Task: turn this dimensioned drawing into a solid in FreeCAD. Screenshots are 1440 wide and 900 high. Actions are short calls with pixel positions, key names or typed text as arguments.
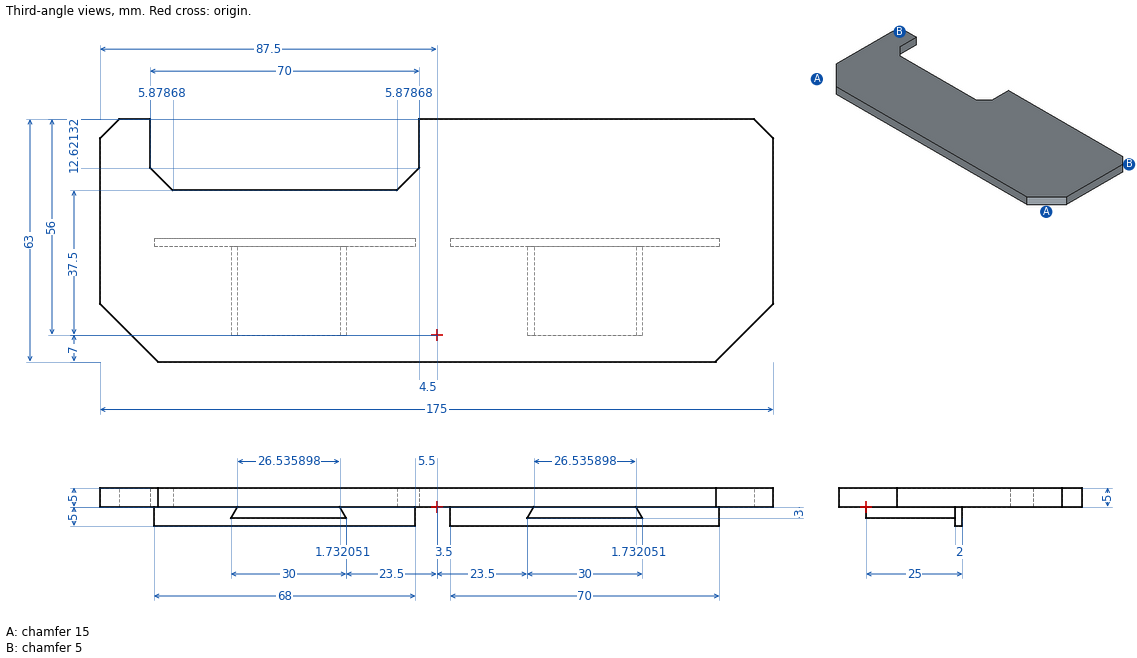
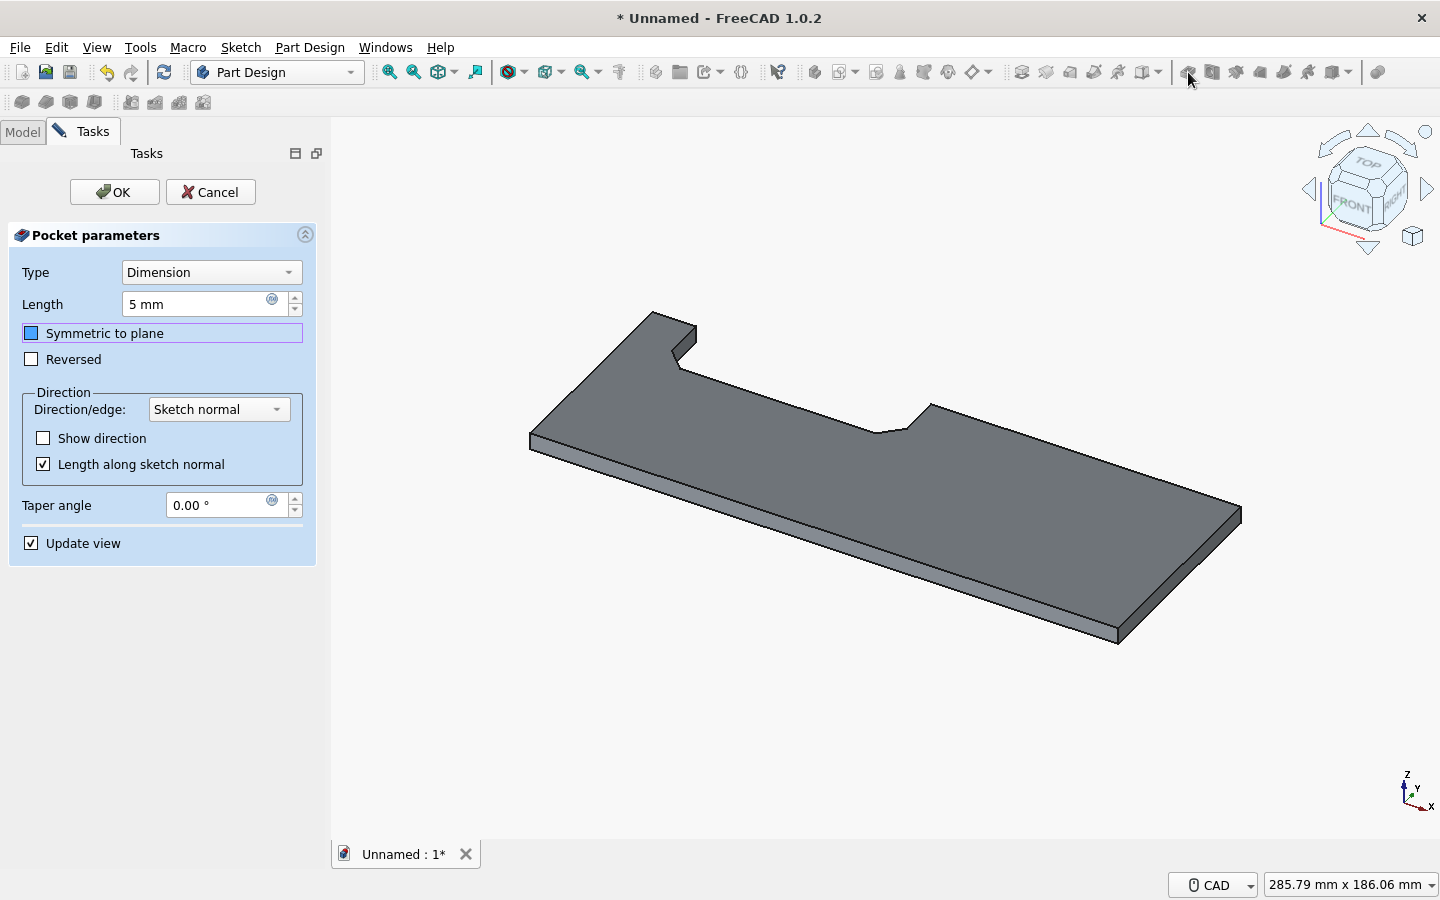
click(115, 192)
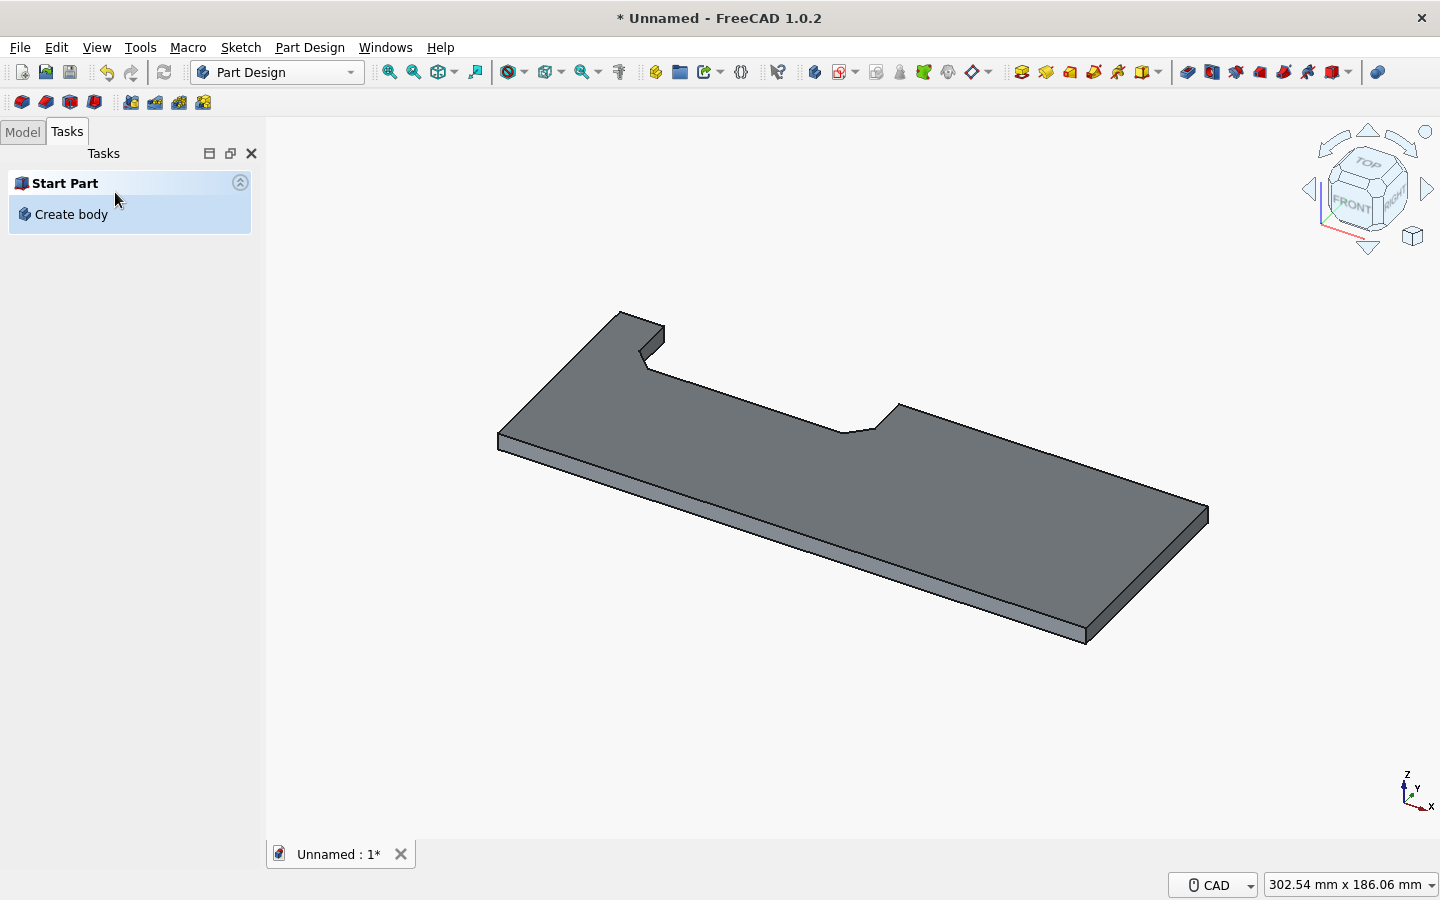
click(1086, 635)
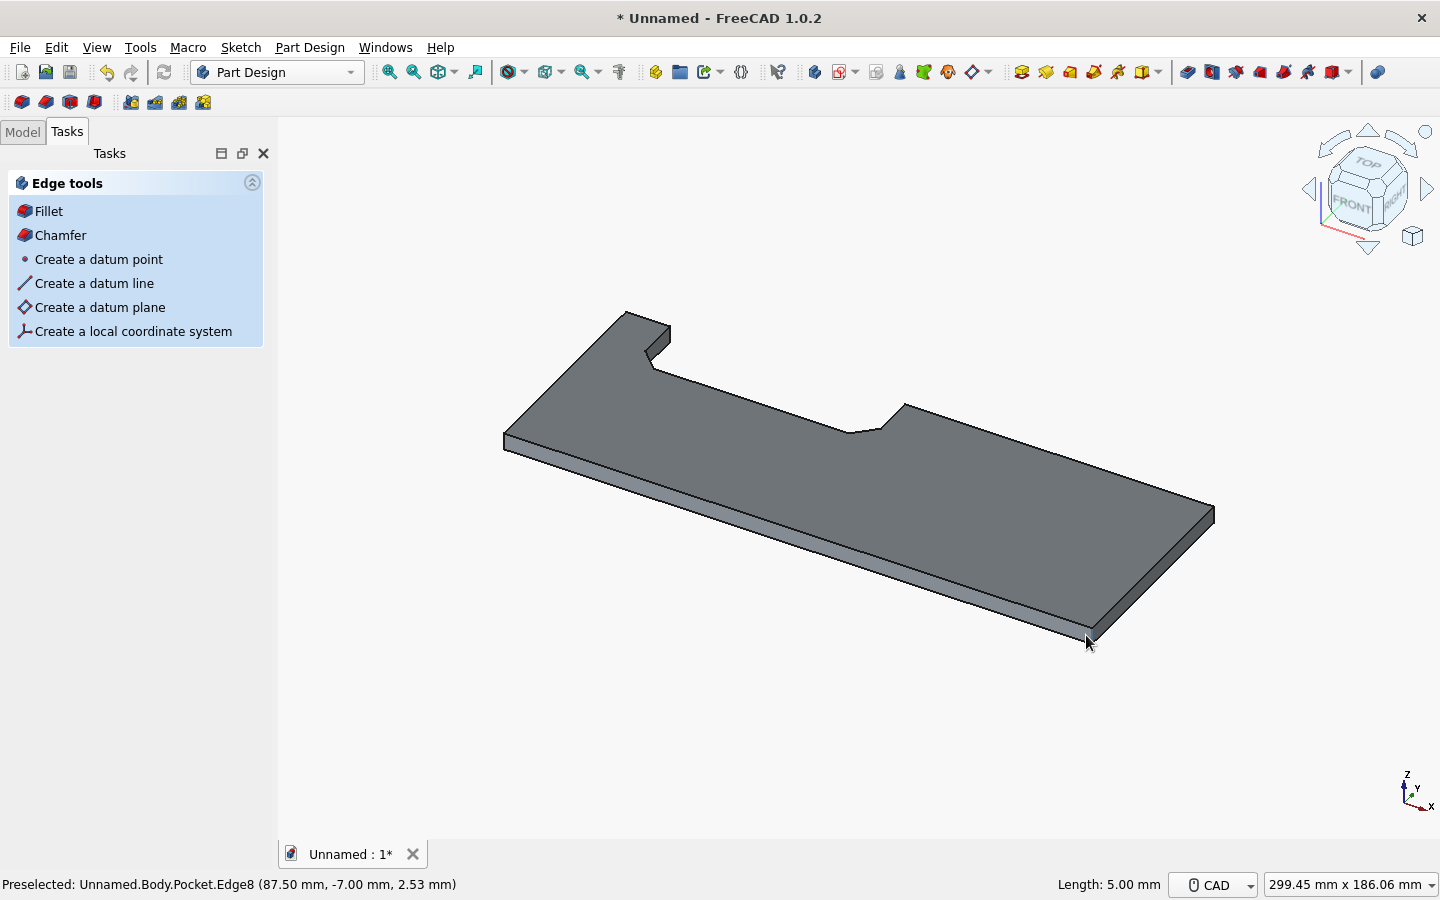
scroll(504, 440, up, 4)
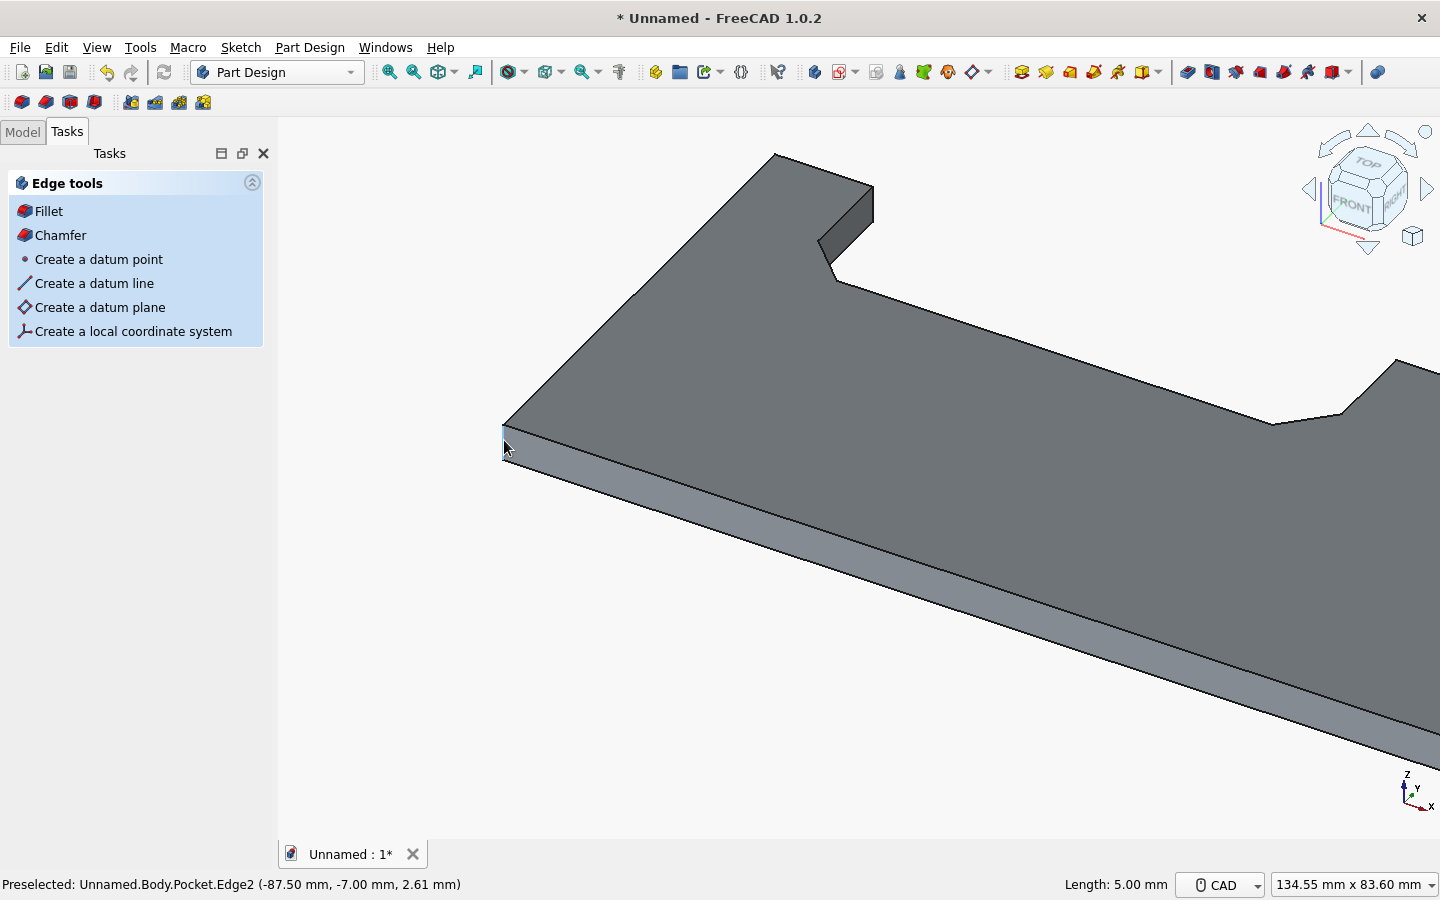
click(390, 72)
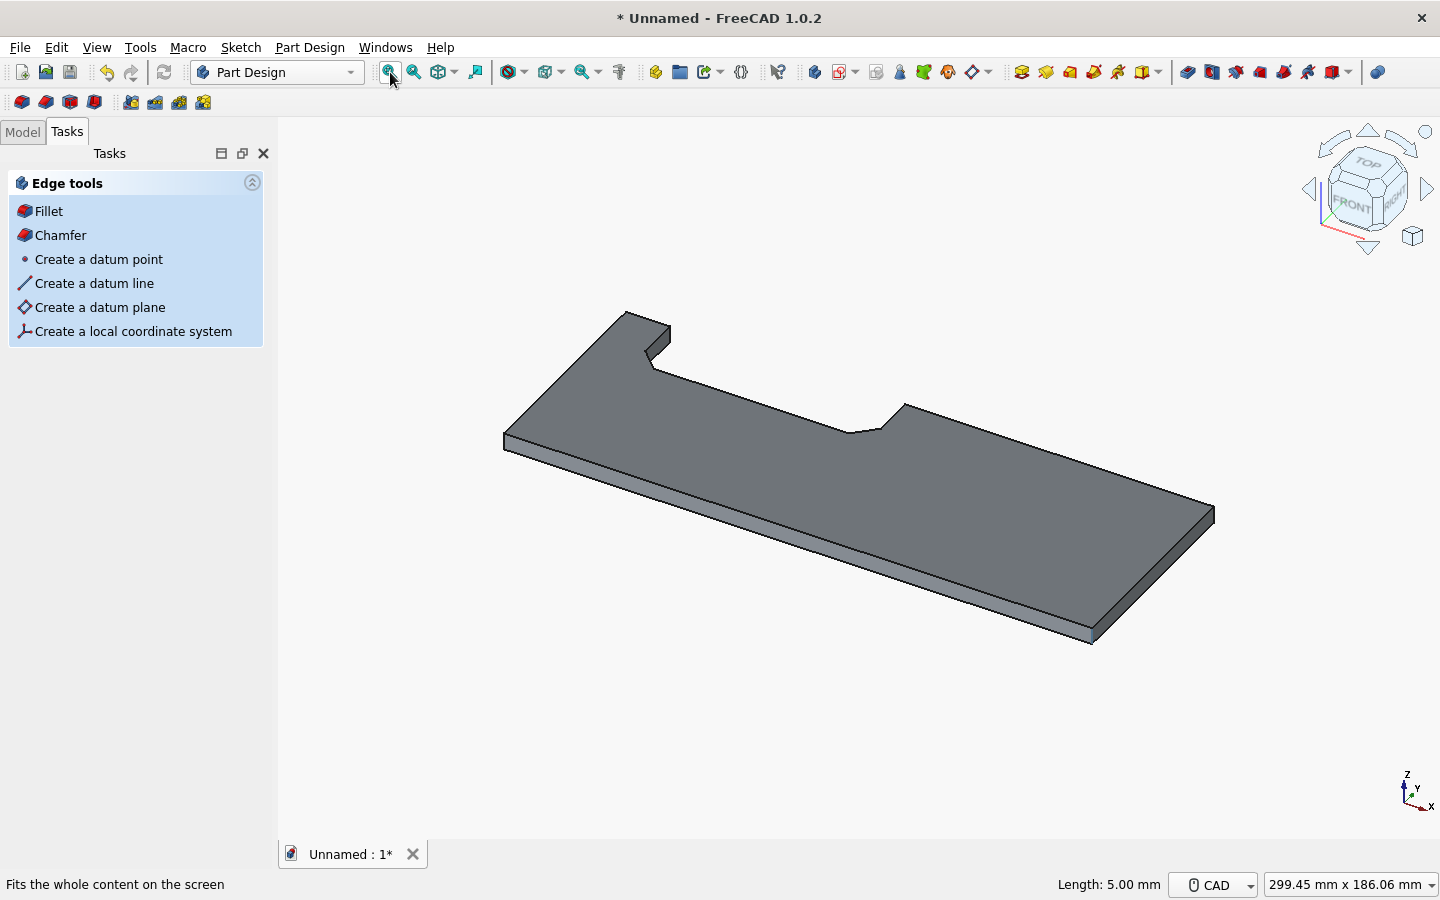
key(0)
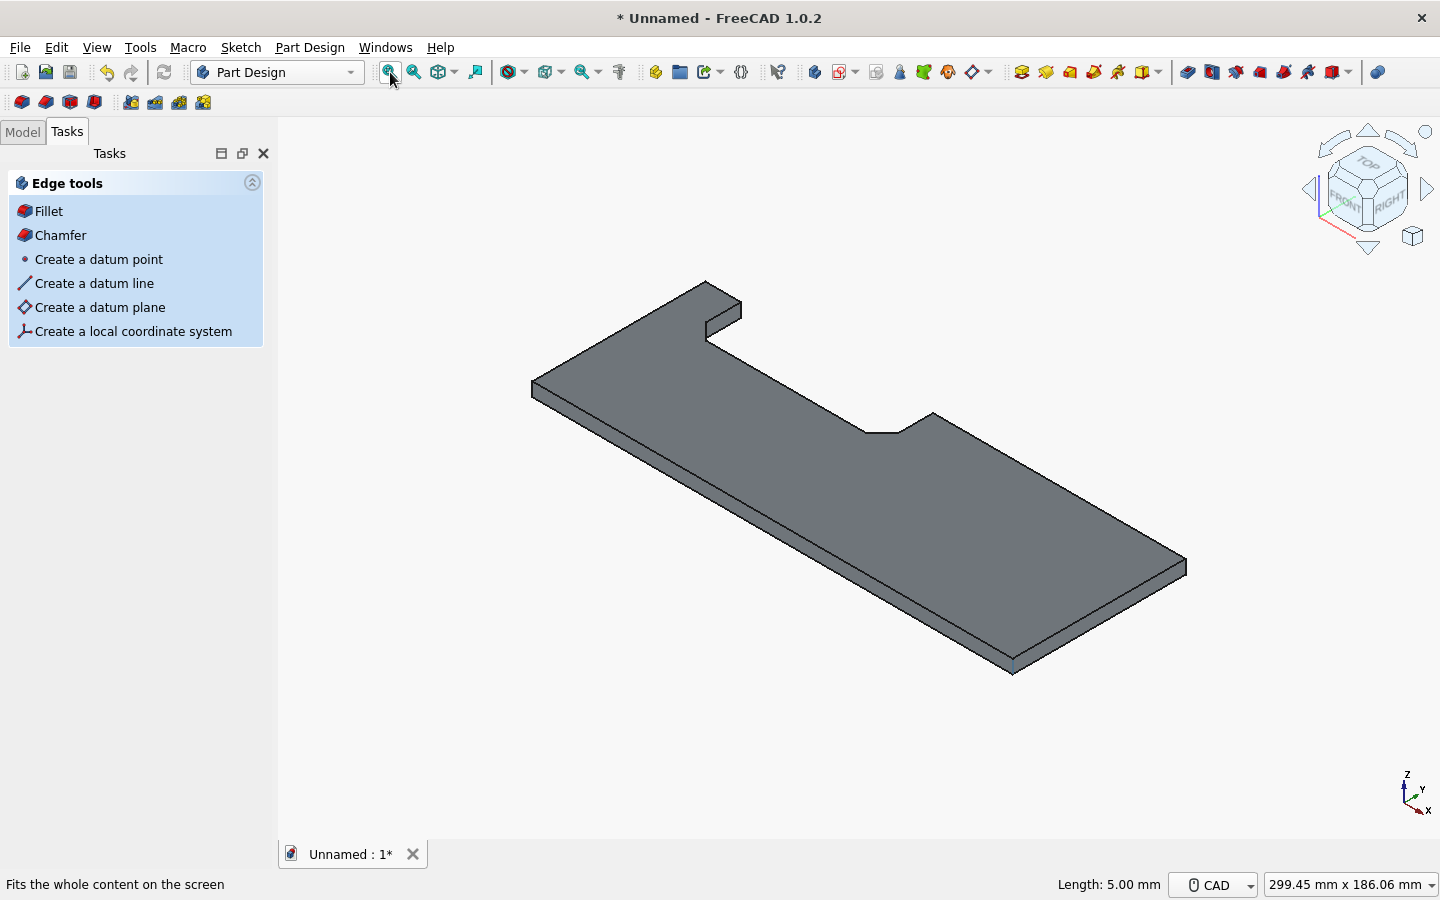
scroll(532, 388, up, 4)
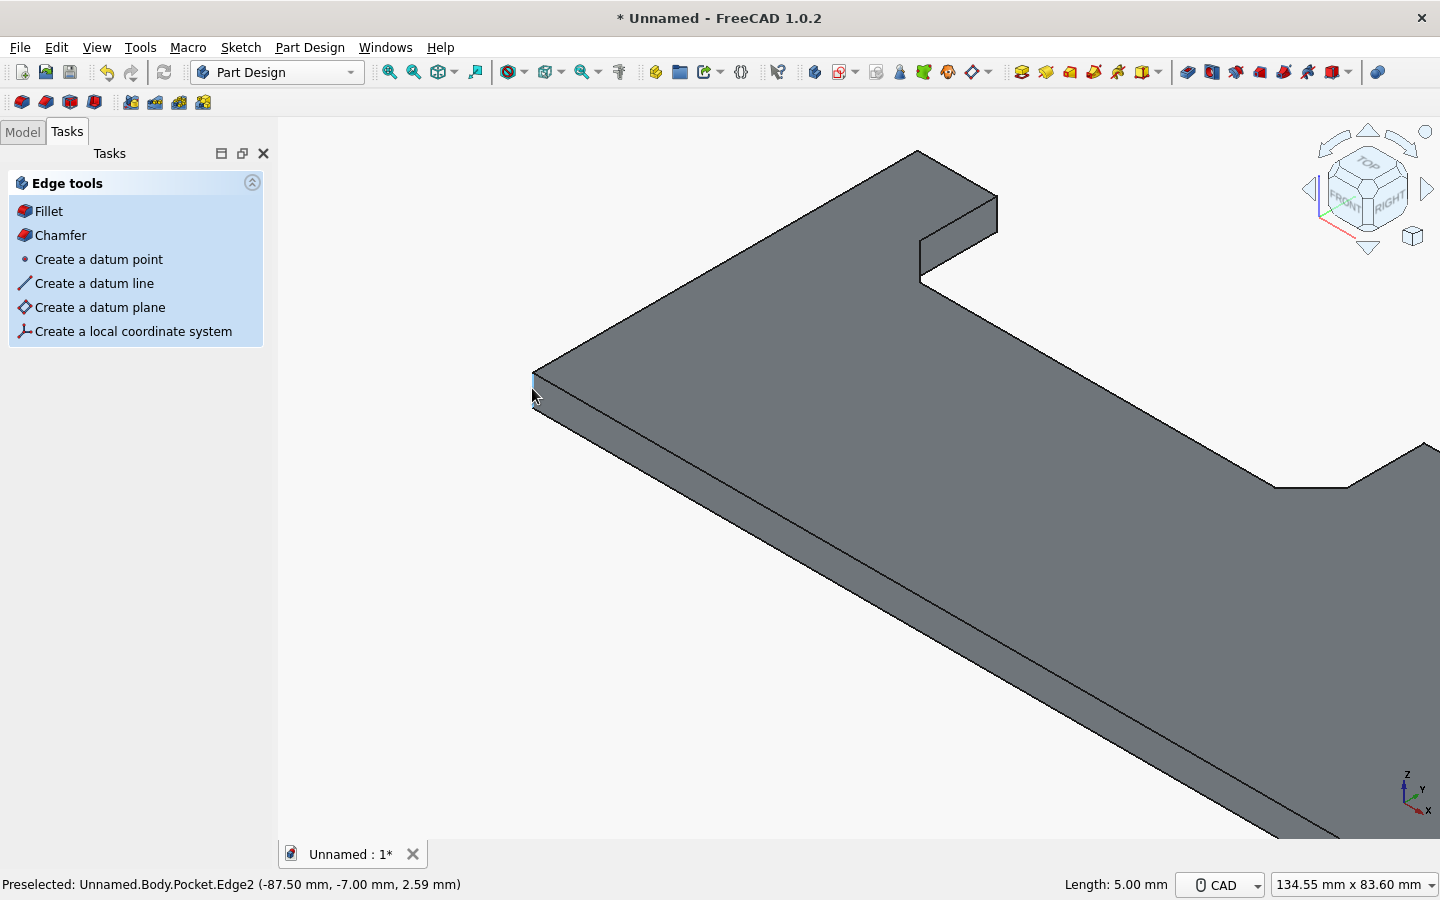
click(390, 72)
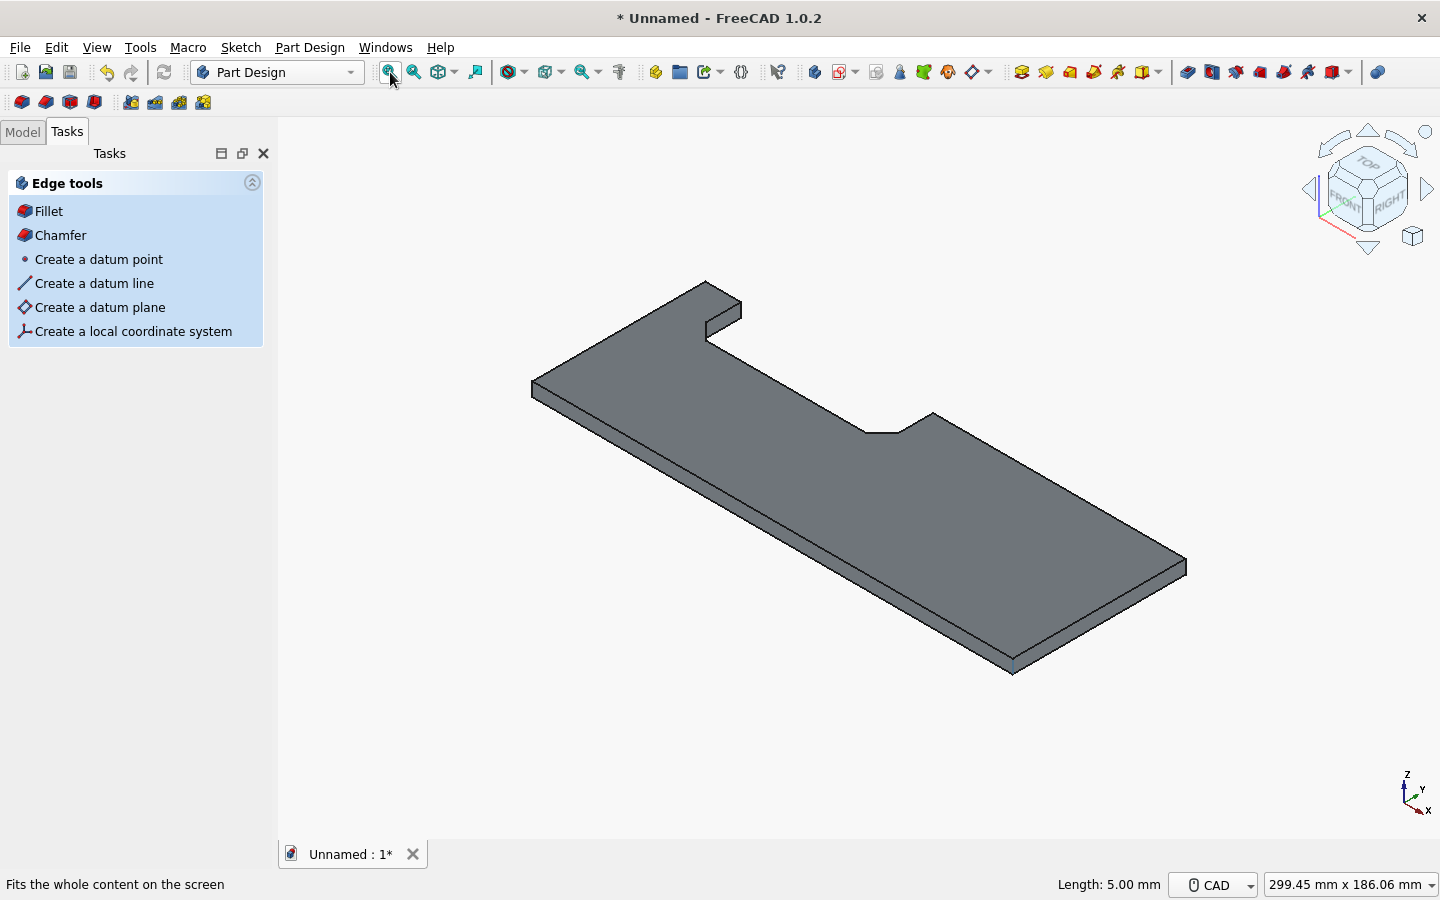
key(2)